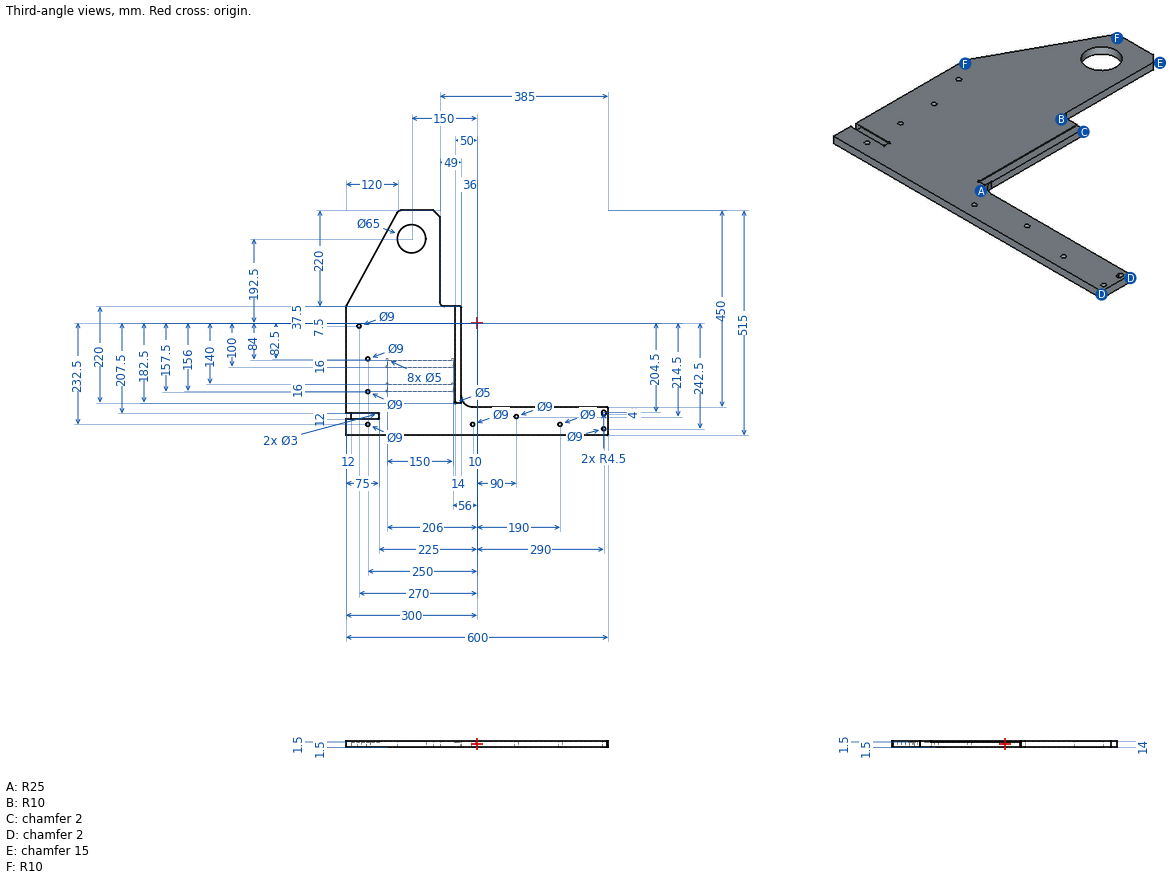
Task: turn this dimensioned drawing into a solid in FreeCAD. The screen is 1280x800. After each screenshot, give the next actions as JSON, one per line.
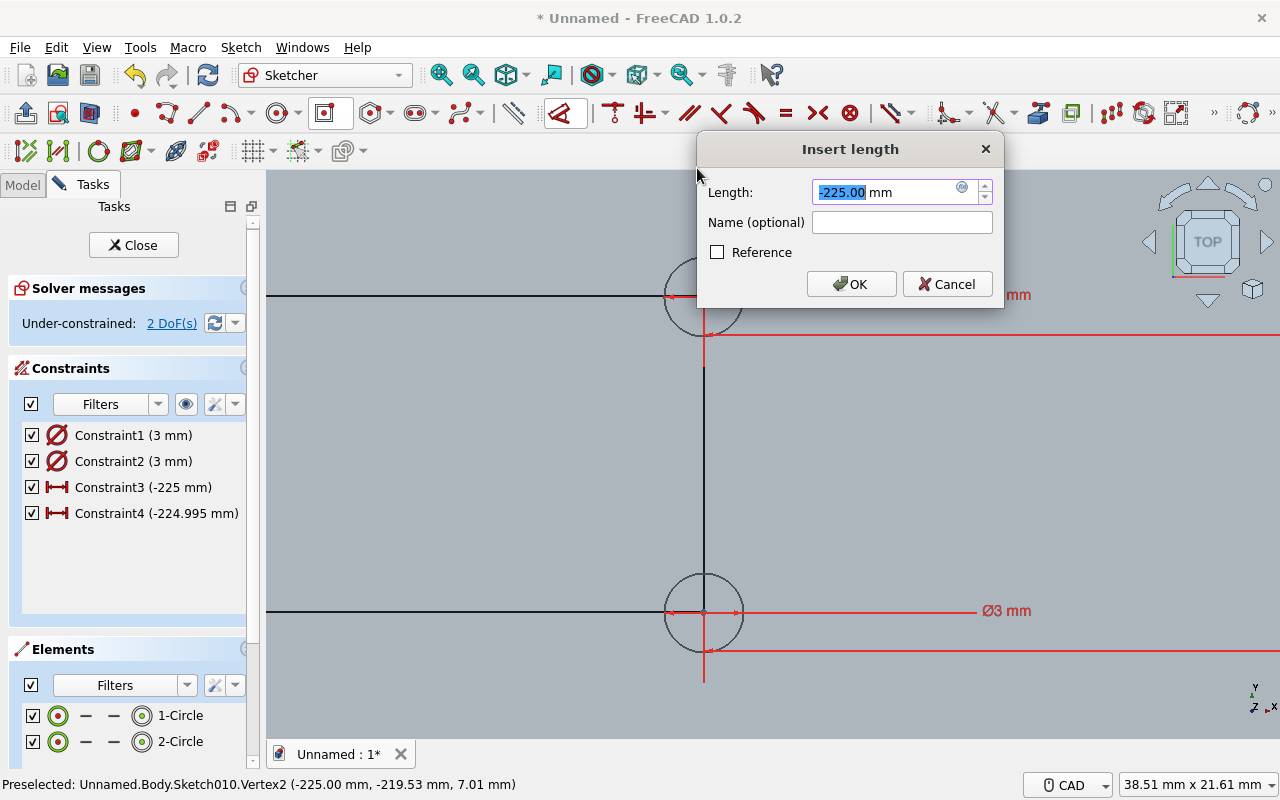
{"action": "type", "text": "-225"}
{"action": "key", "text": "Return"}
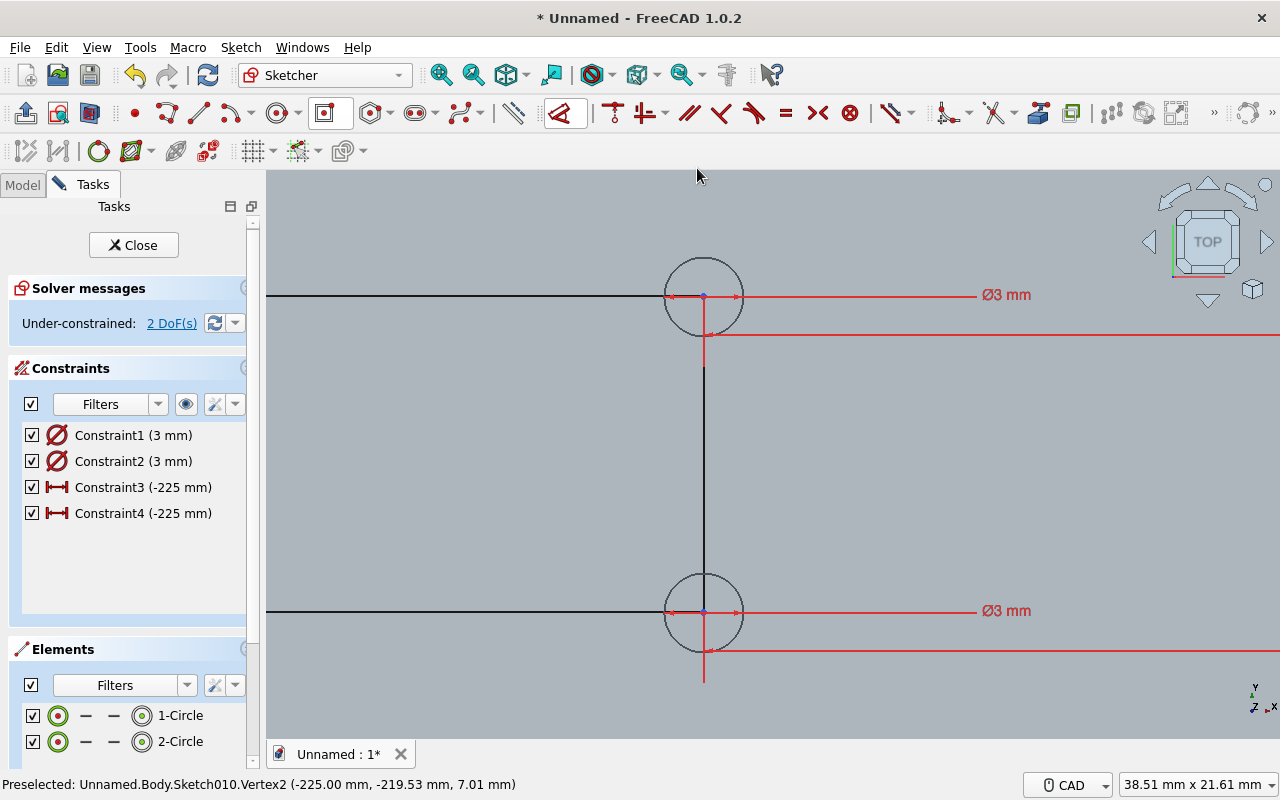
{"action": "left_click", "coordinate": [704, 297]}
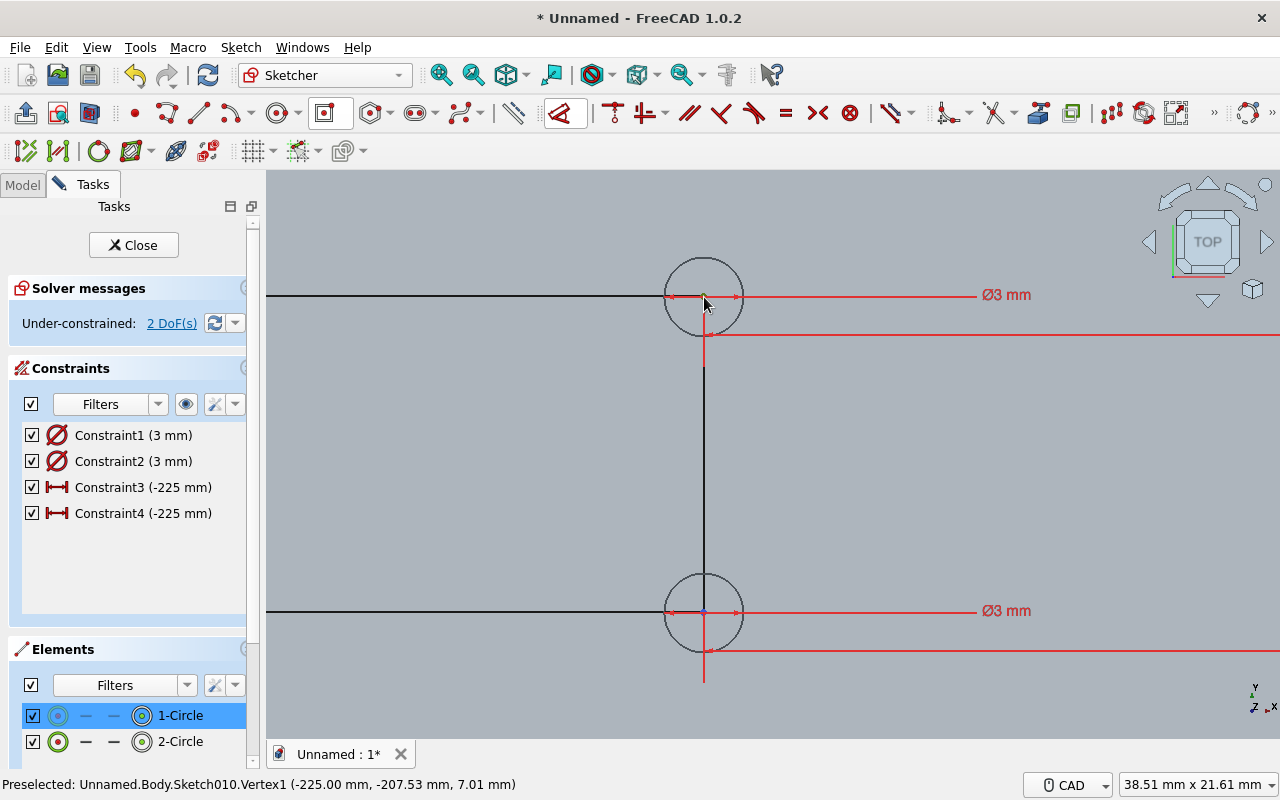
{"action": "left_click", "coordinate": [704, 613]}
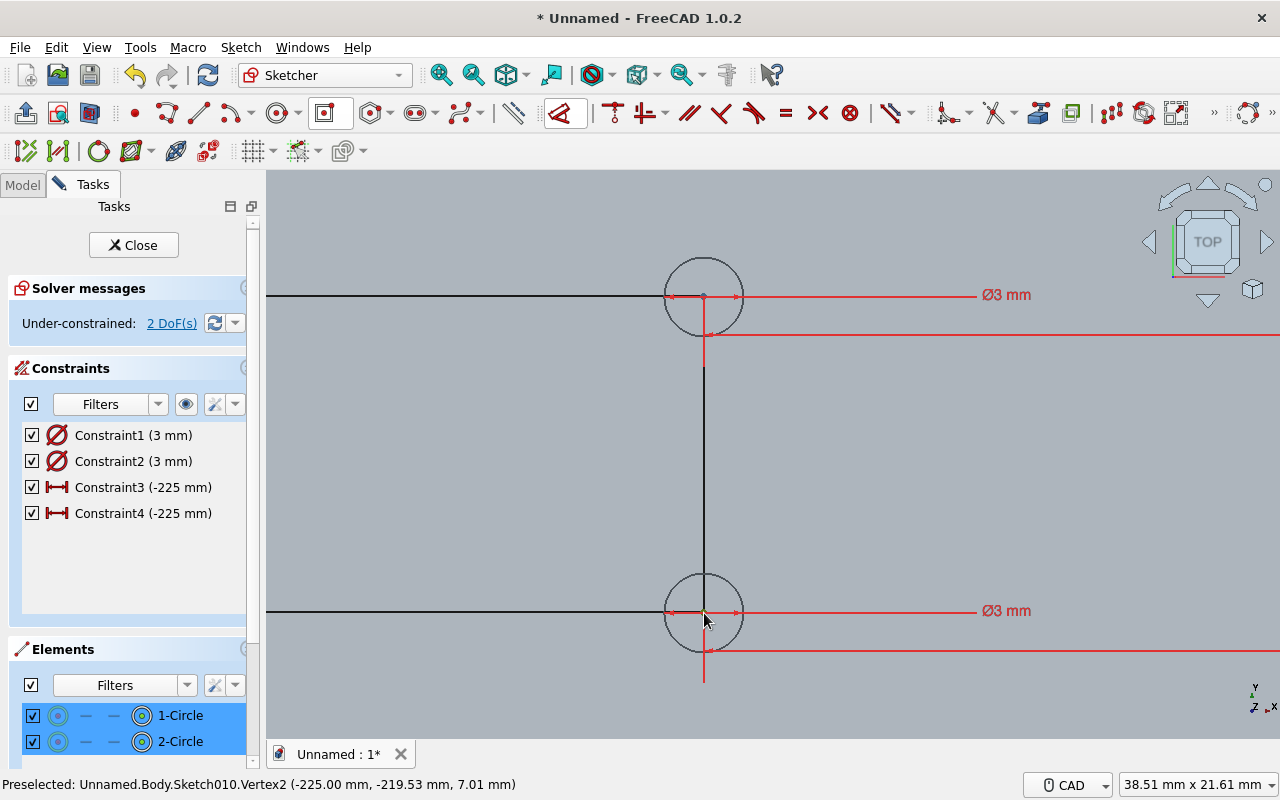
{"action": "key", "text": "i"}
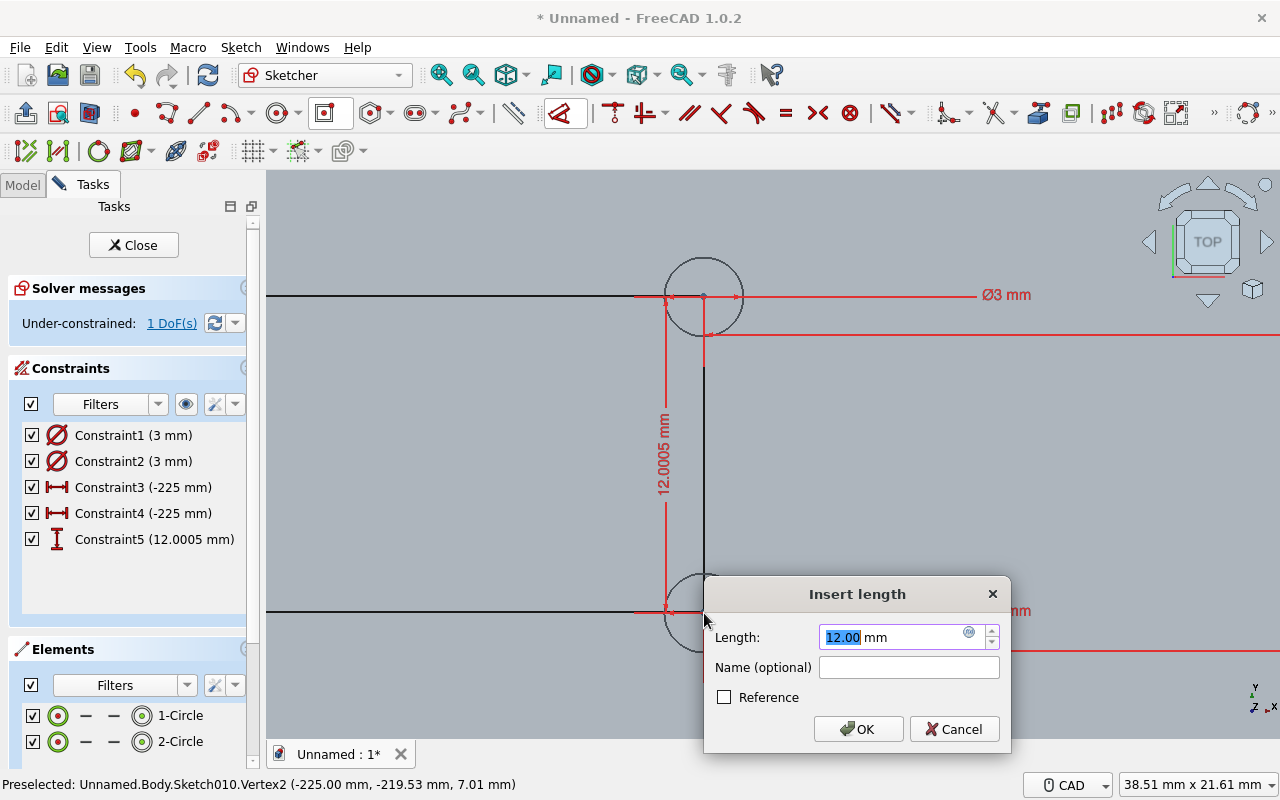
{"action": "type", "text": "12"}
{"action": "key", "text": "Return"}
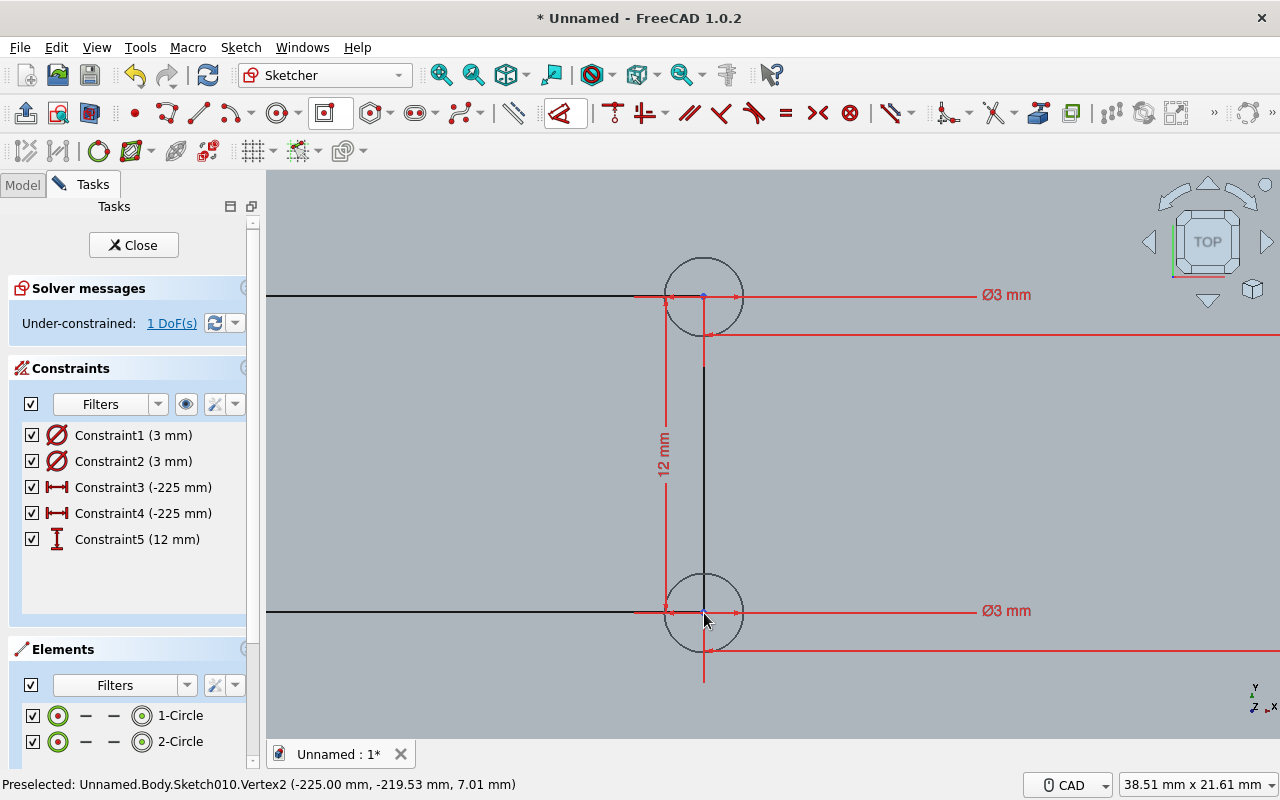
{"action": "left_click", "coordinate": [704, 297]}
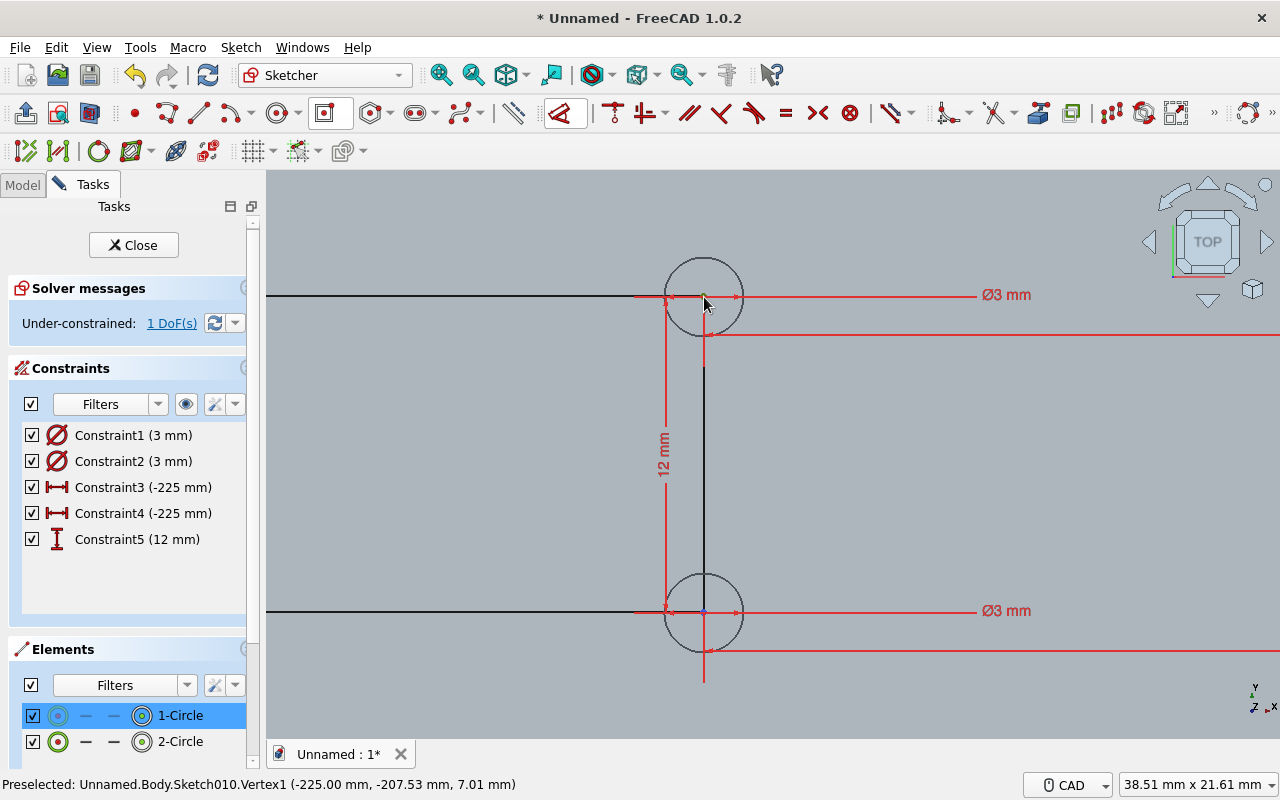
{"action": "left_click", "coordinate": [582, 114]}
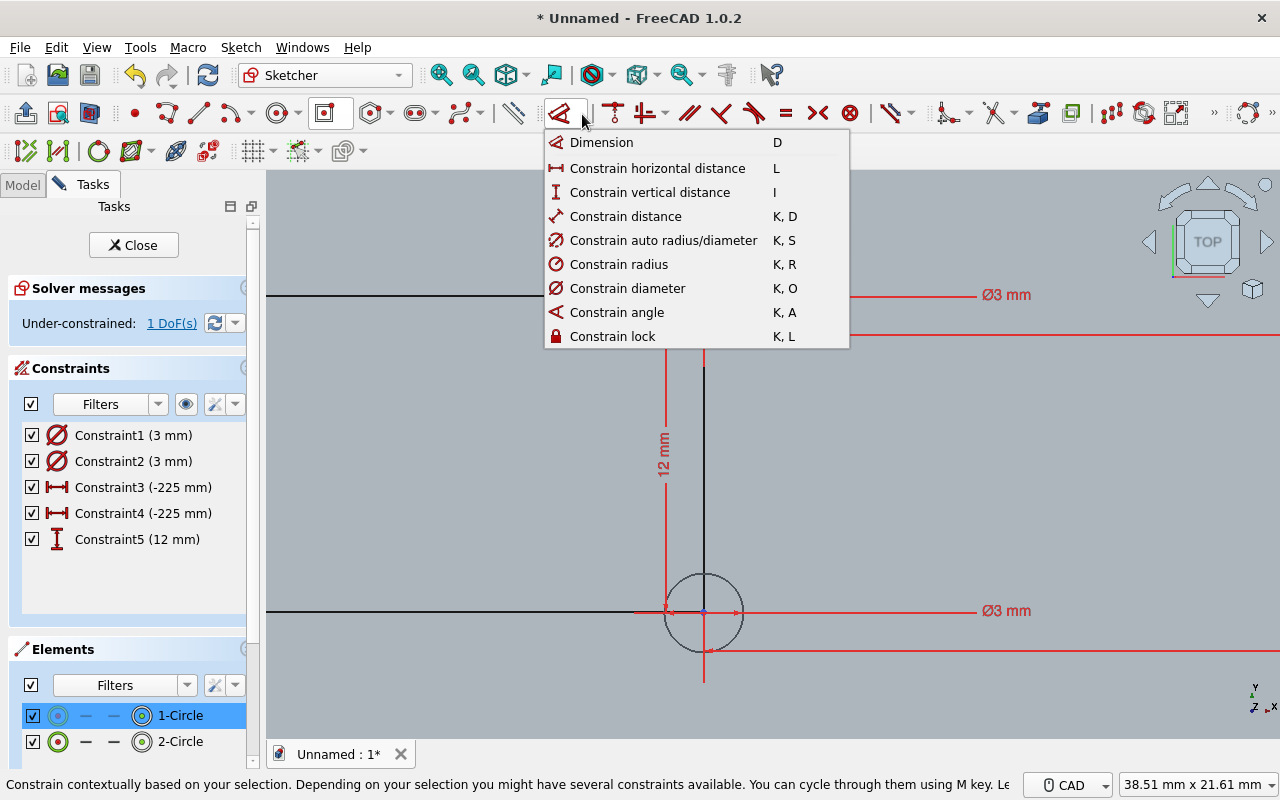
{"action": "left_click", "coordinate": [697, 192]}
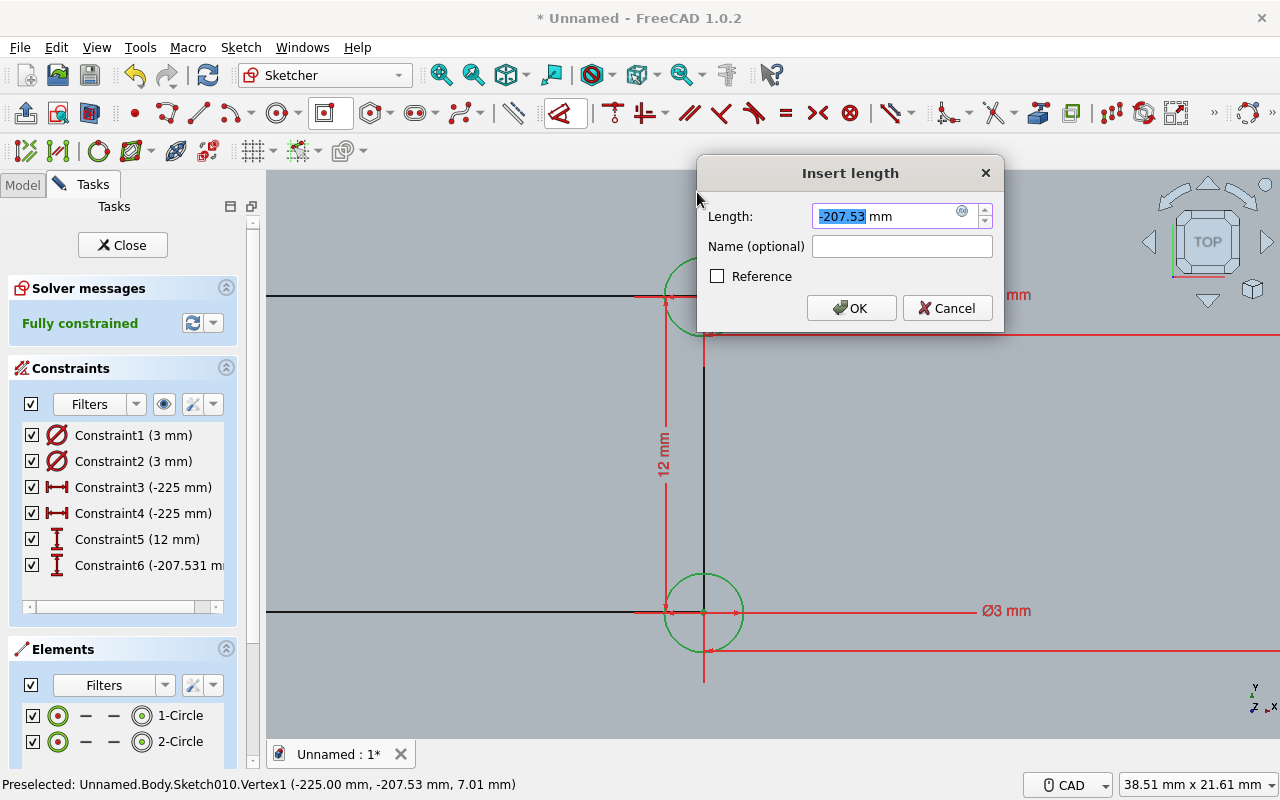
{"action": "type", "text": "-207.5"}
{"action": "key", "text": "Return"}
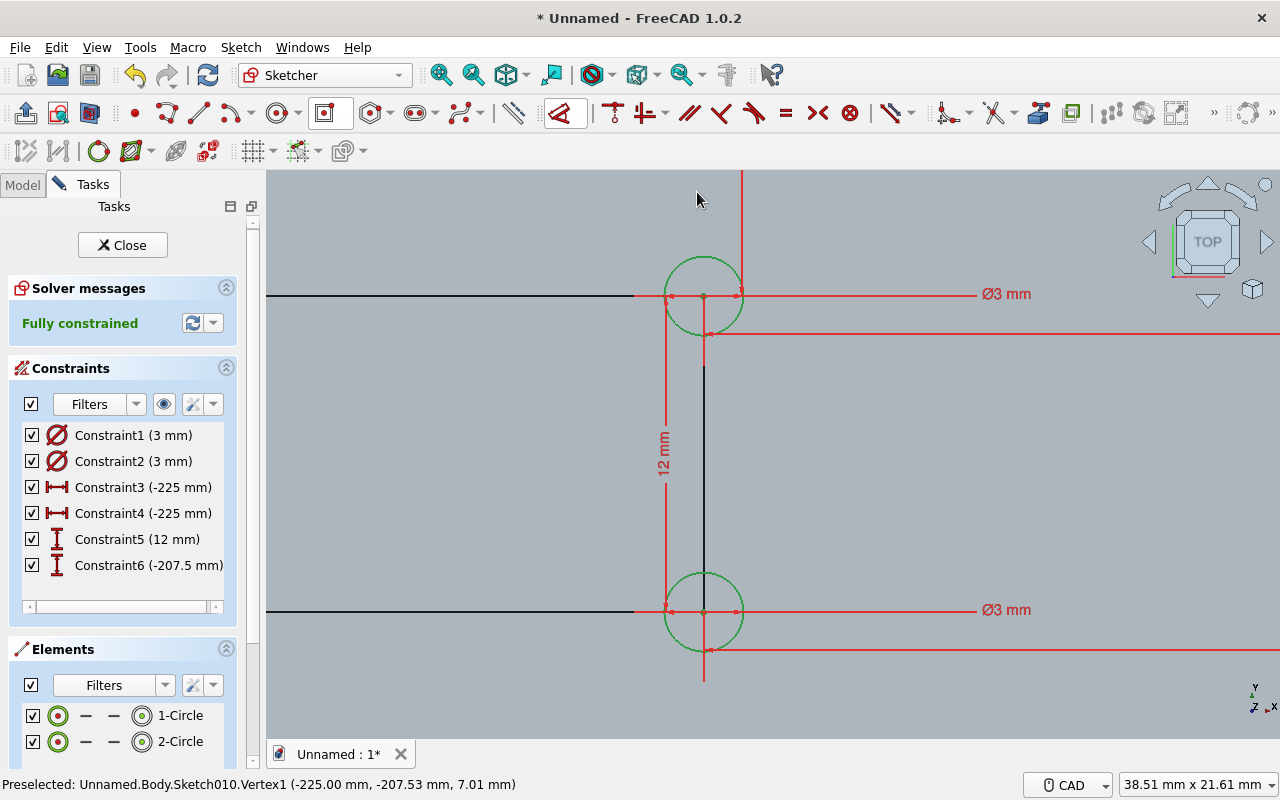
{"action": "left_click", "coordinate": [123, 245]}